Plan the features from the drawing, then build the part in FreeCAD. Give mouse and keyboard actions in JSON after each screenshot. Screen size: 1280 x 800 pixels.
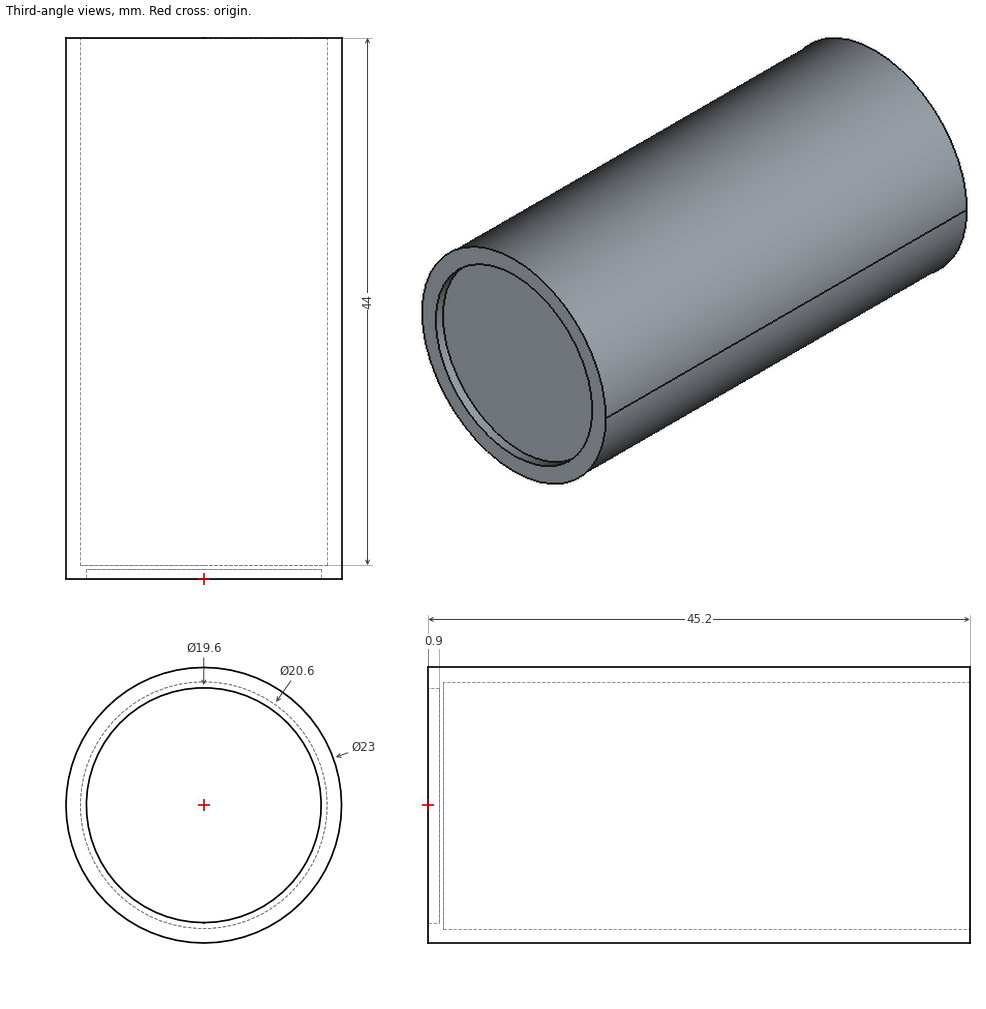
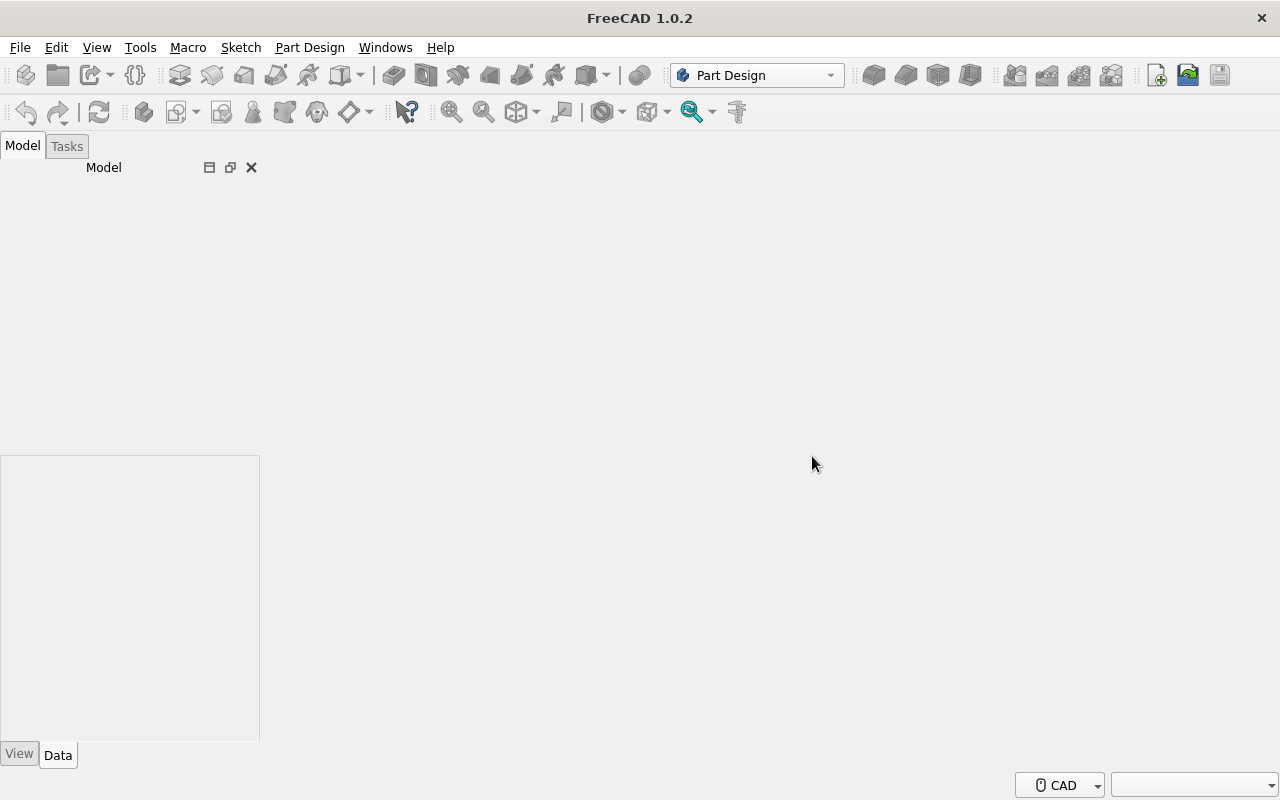
{"action": "left_click", "coordinate": [1156, 76]}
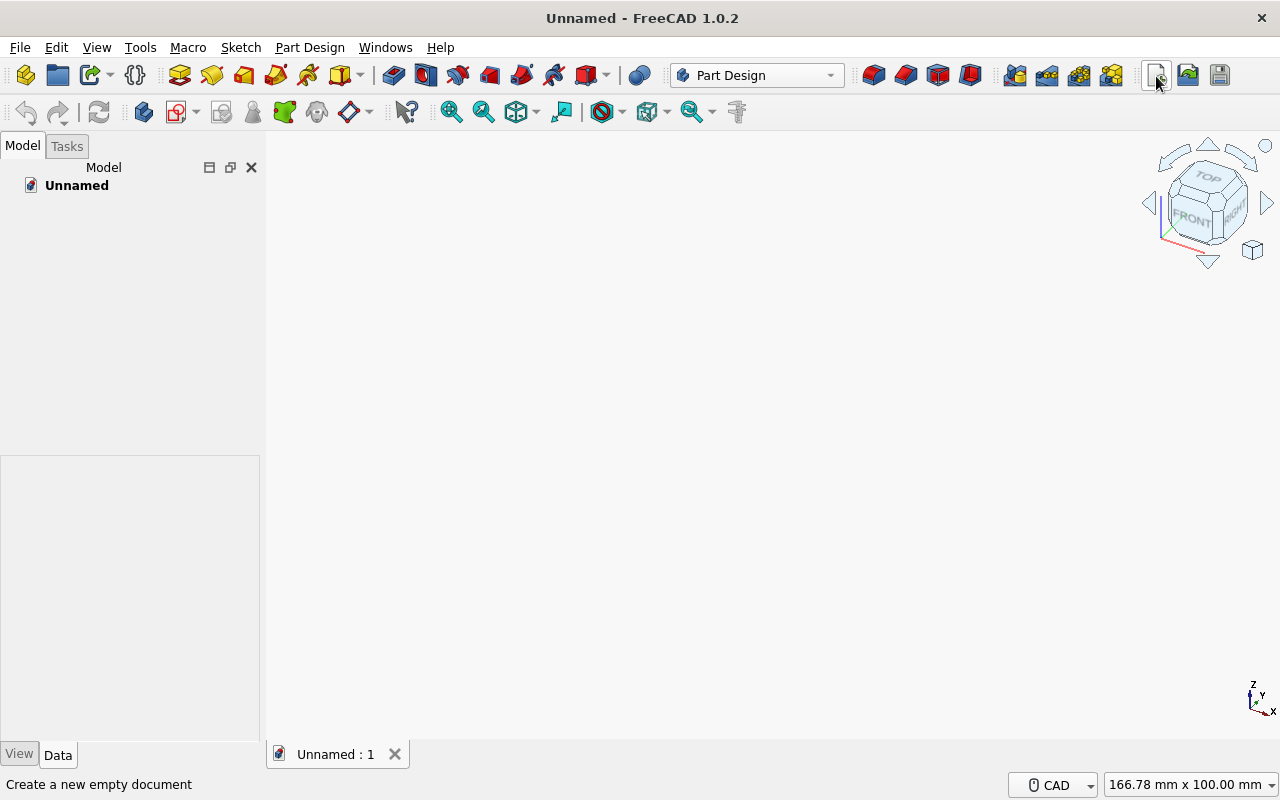
{"action": "left_click", "coordinate": [176, 112]}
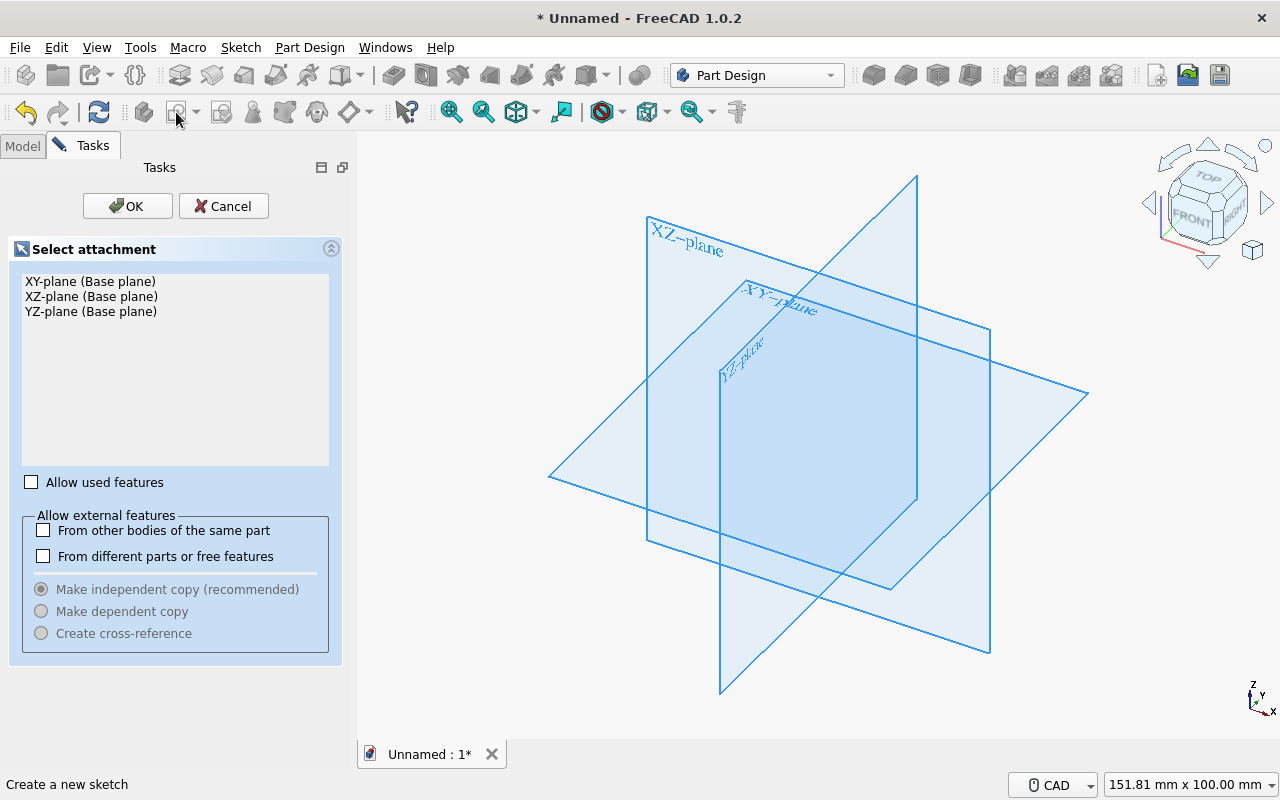
{"action": "left_click", "coordinate": [82, 296]}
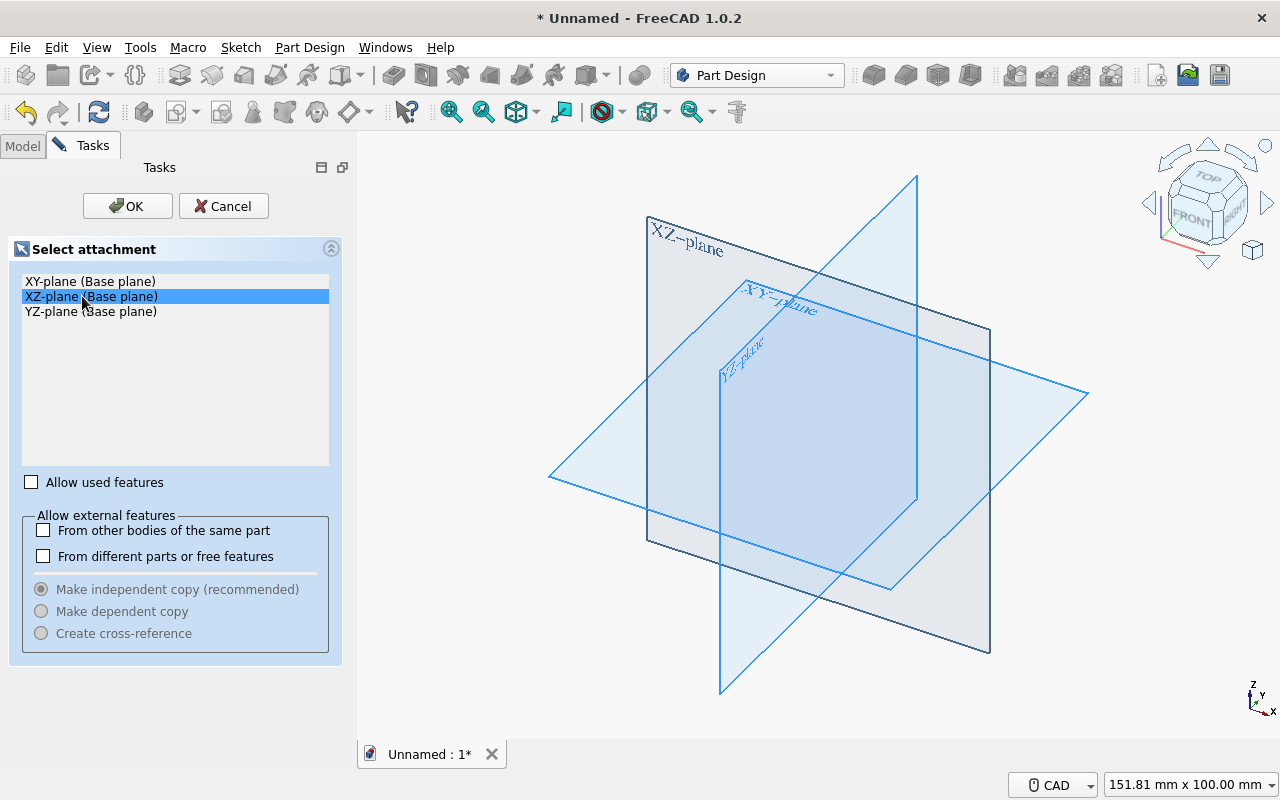
{"action": "left_click", "coordinate": [128, 206]}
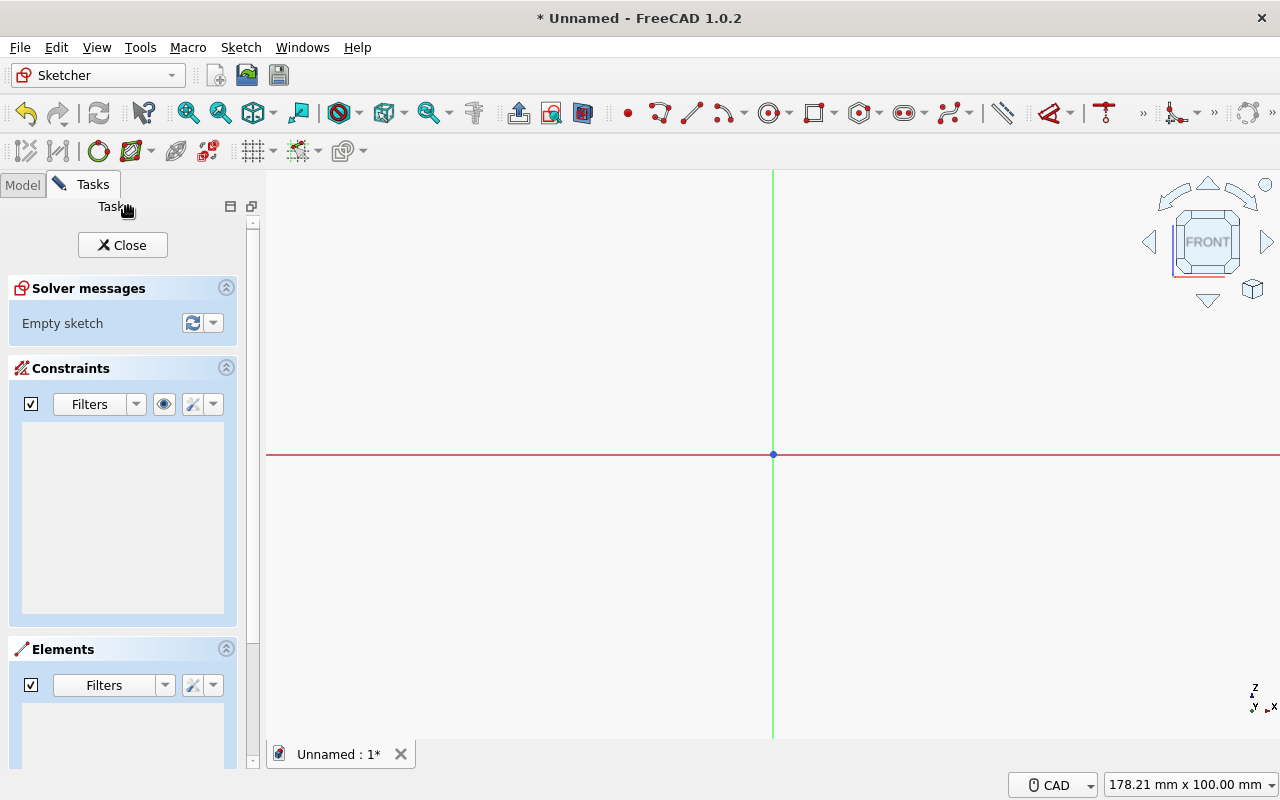
{"action": "scroll", "coordinate": [813, 454], "scroll_direction": "up", "scroll_amount": 5}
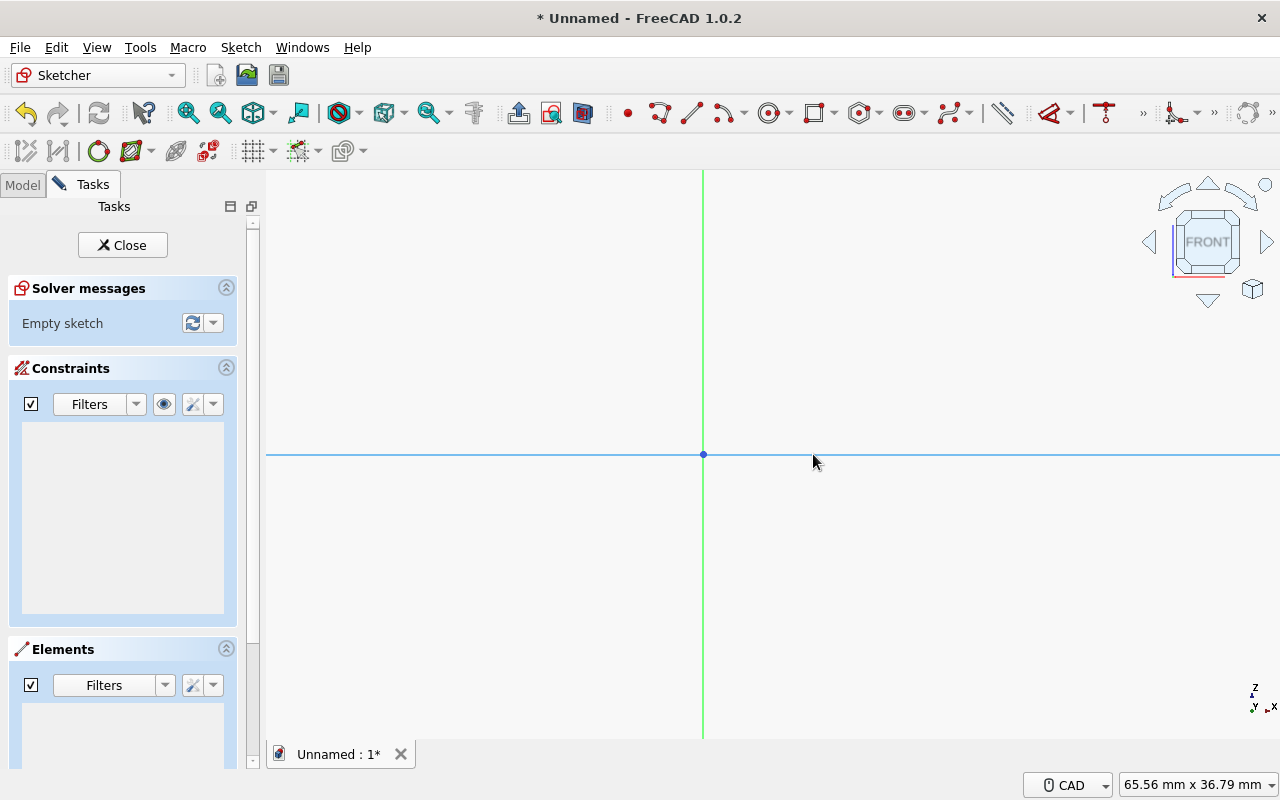
{"action": "left_click", "coordinate": [770, 114]}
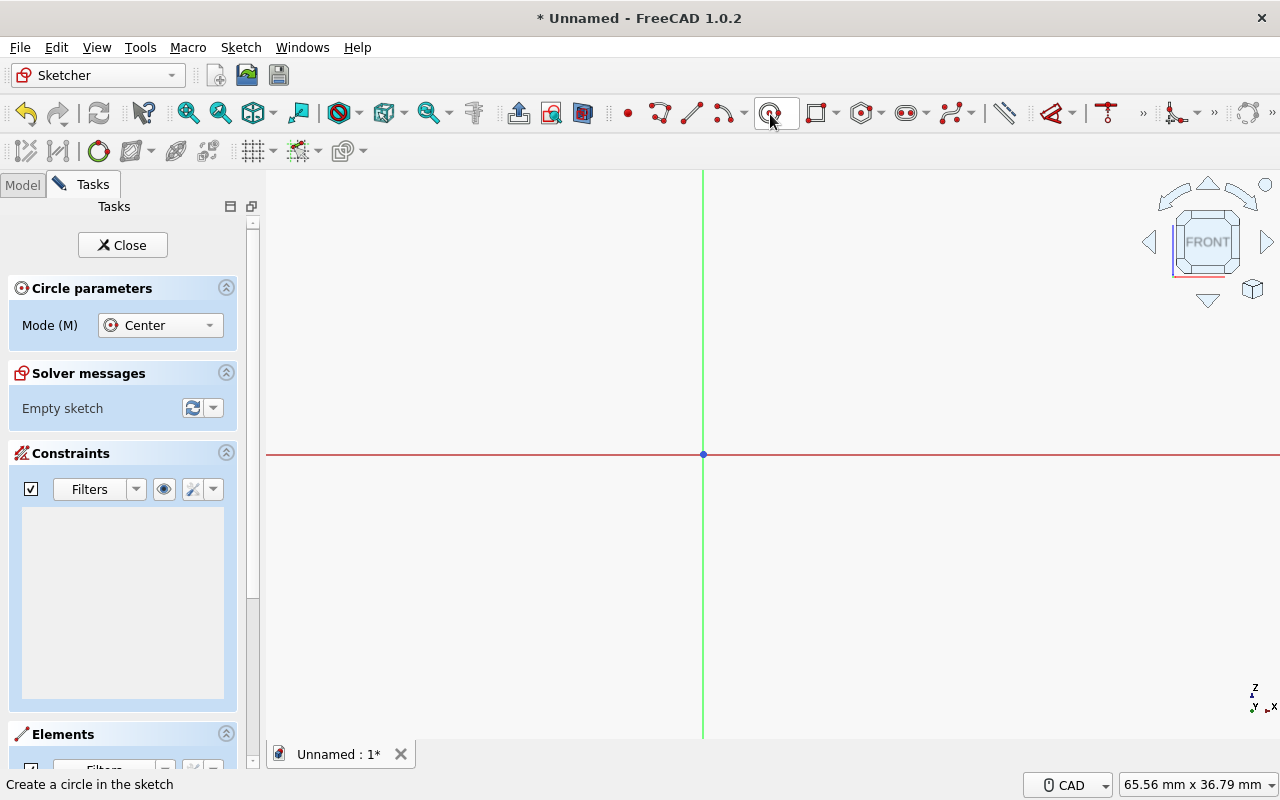
{"action": "left_click", "coordinate": [703, 454]}
{"action": "mouse_move", "coordinate": [829, 329]}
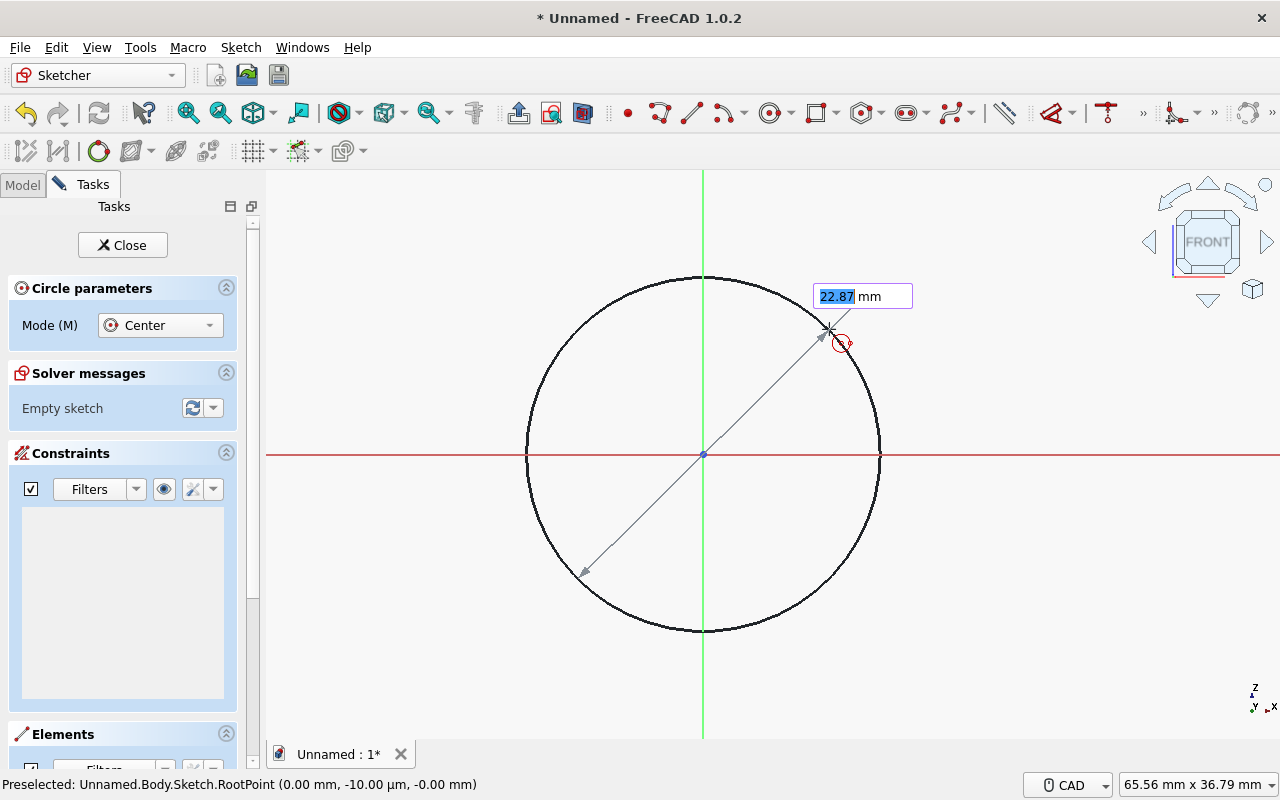
{"action": "type", "text": "23"}
{"action": "key", "text": "Return"}
{"action": "key", "text": "Escape"}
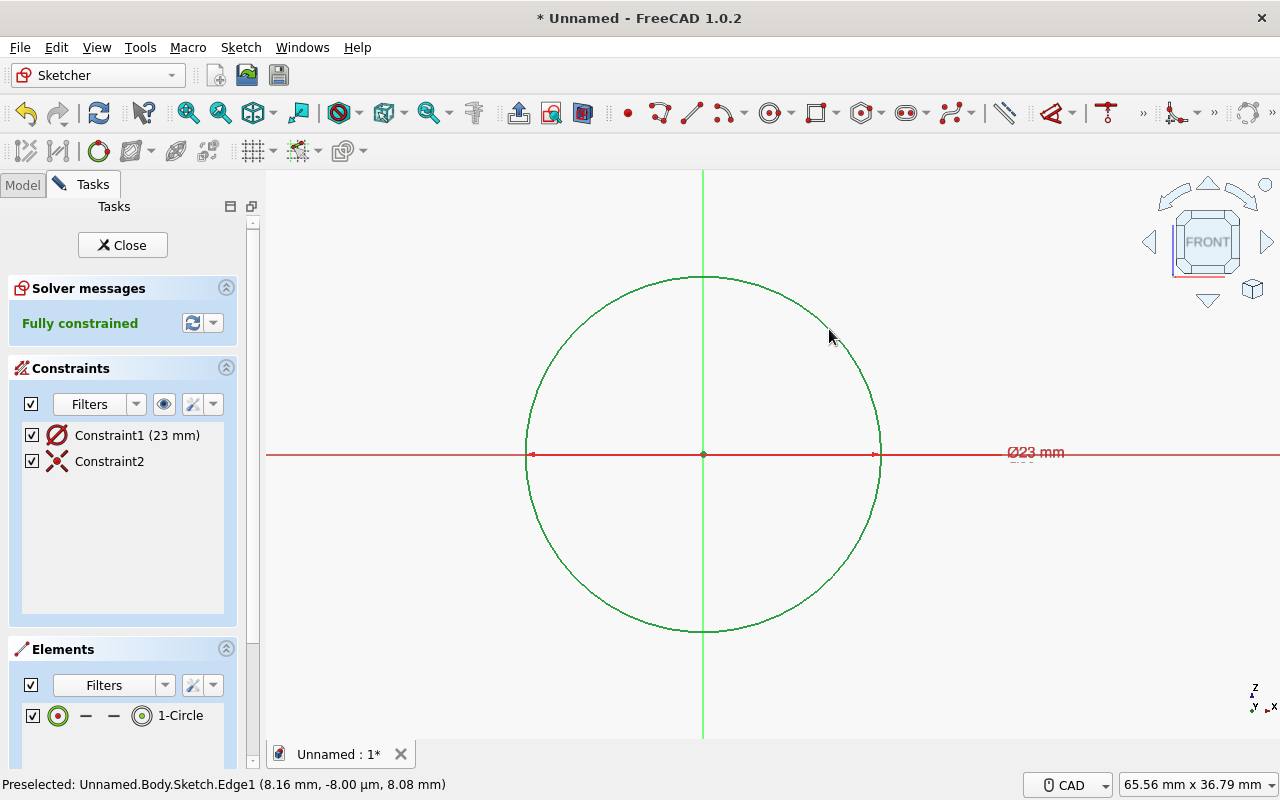
{"action": "left_click", "coordinate": [123, 245]}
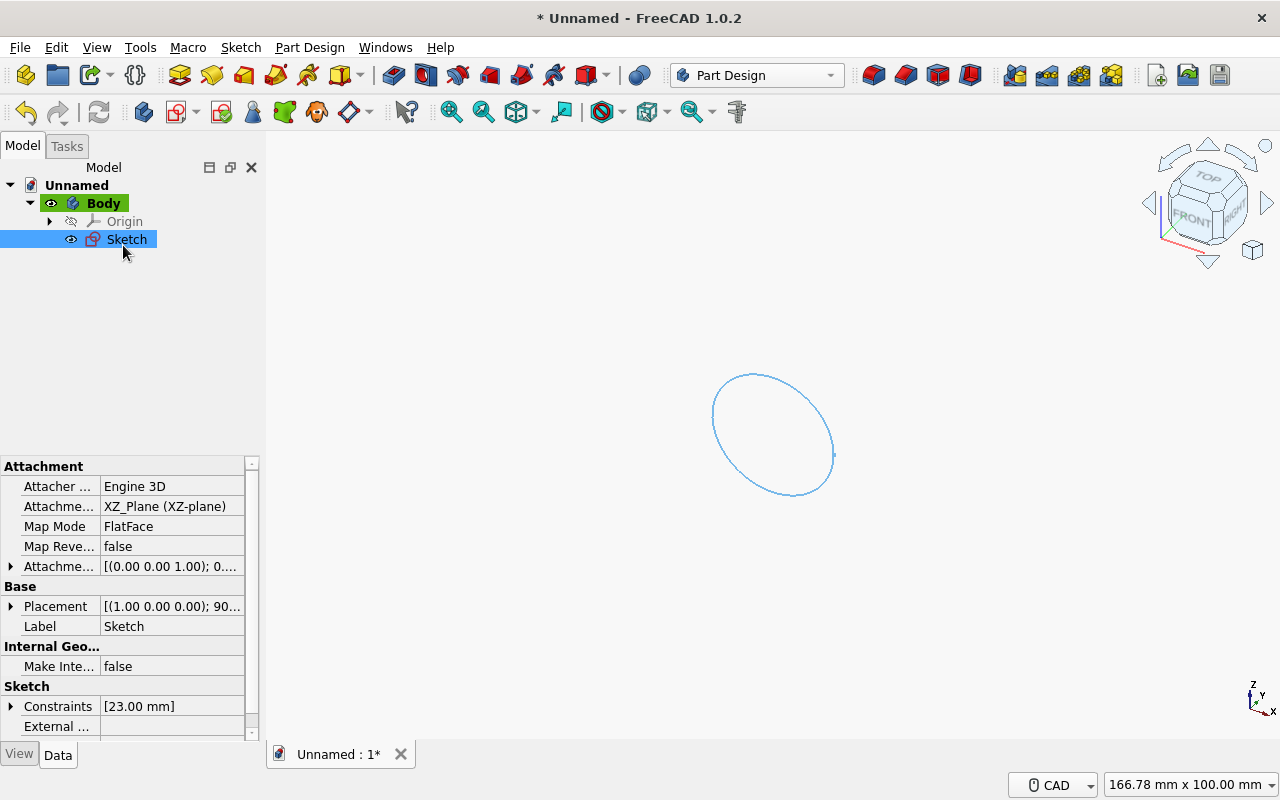
{"action": "left_click", "coordinate": [180, 76]}